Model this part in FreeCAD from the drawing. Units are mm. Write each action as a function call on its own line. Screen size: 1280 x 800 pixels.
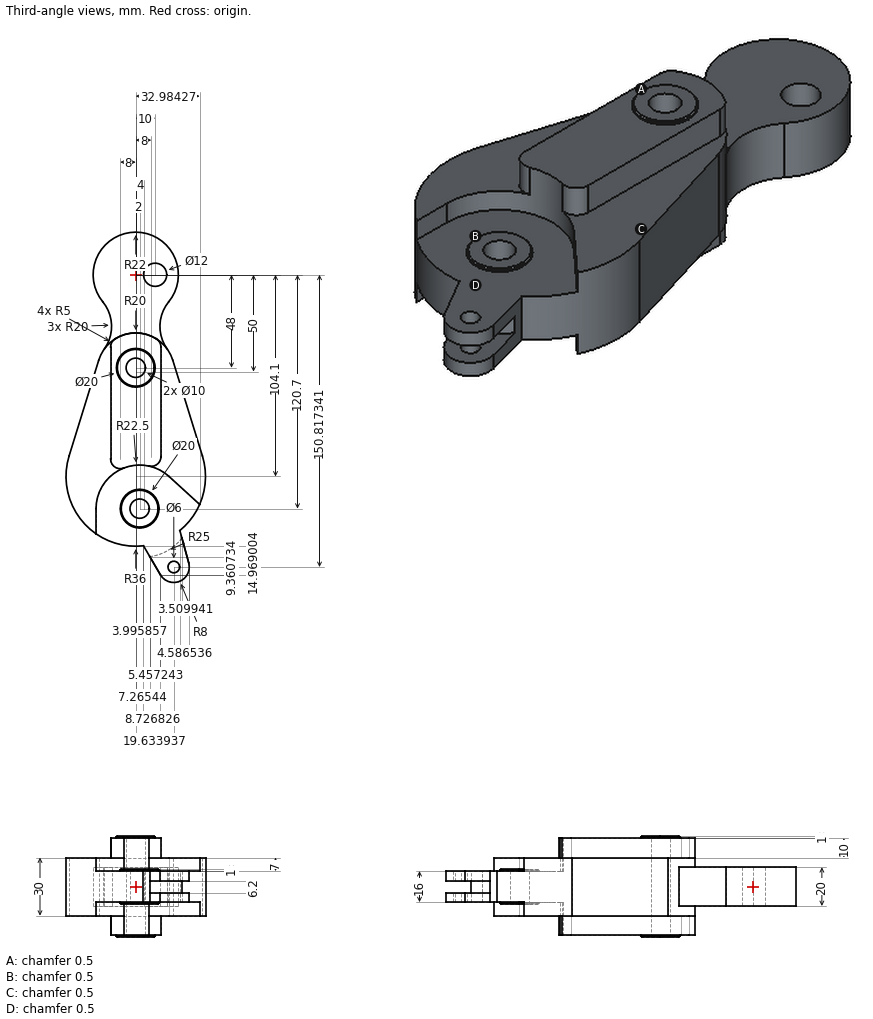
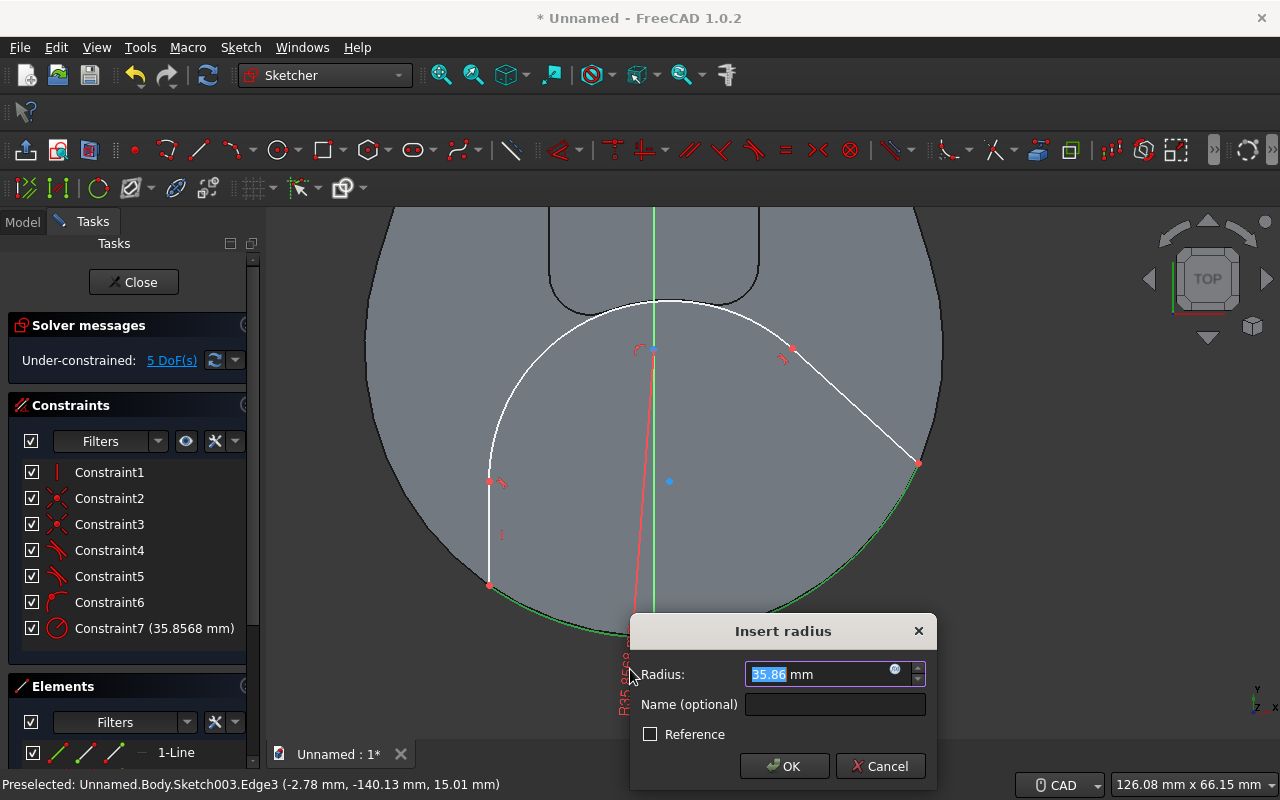
text(36)
key(Return)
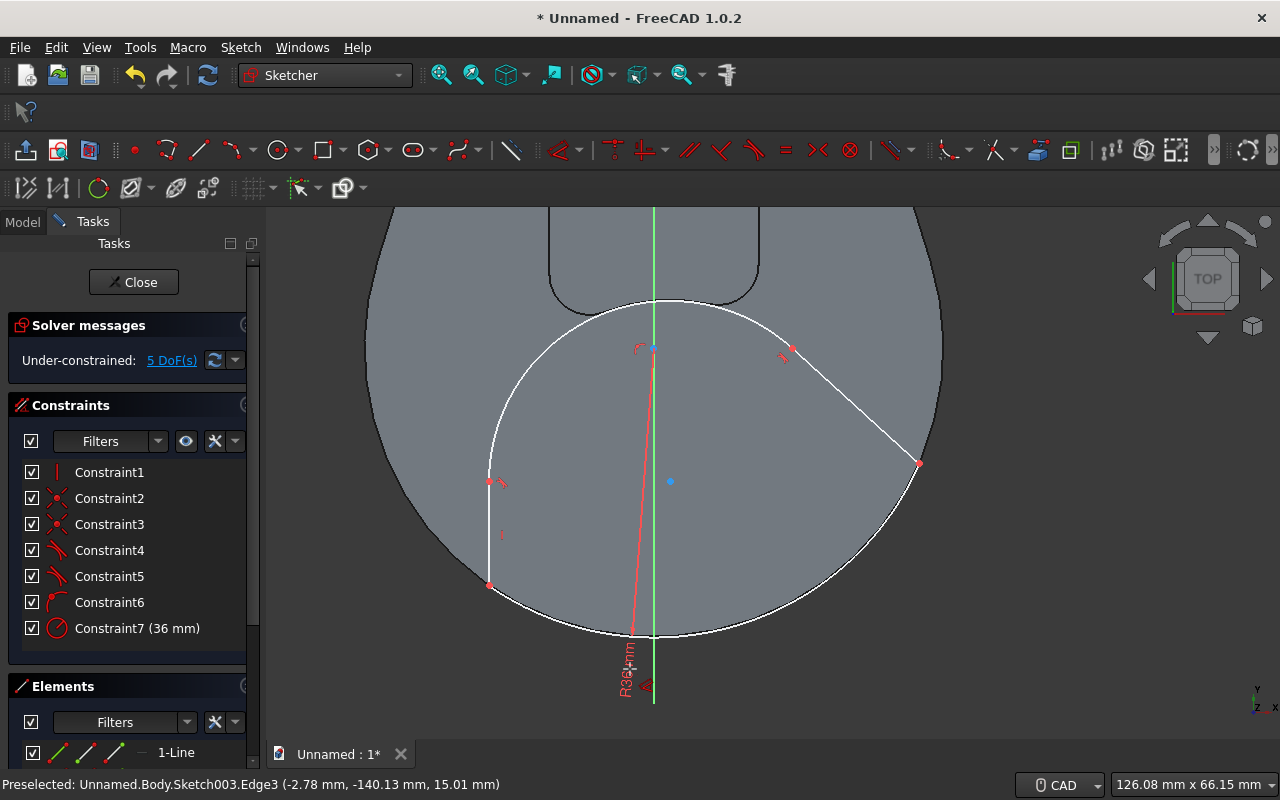
click(678, 301)
click(679, 269)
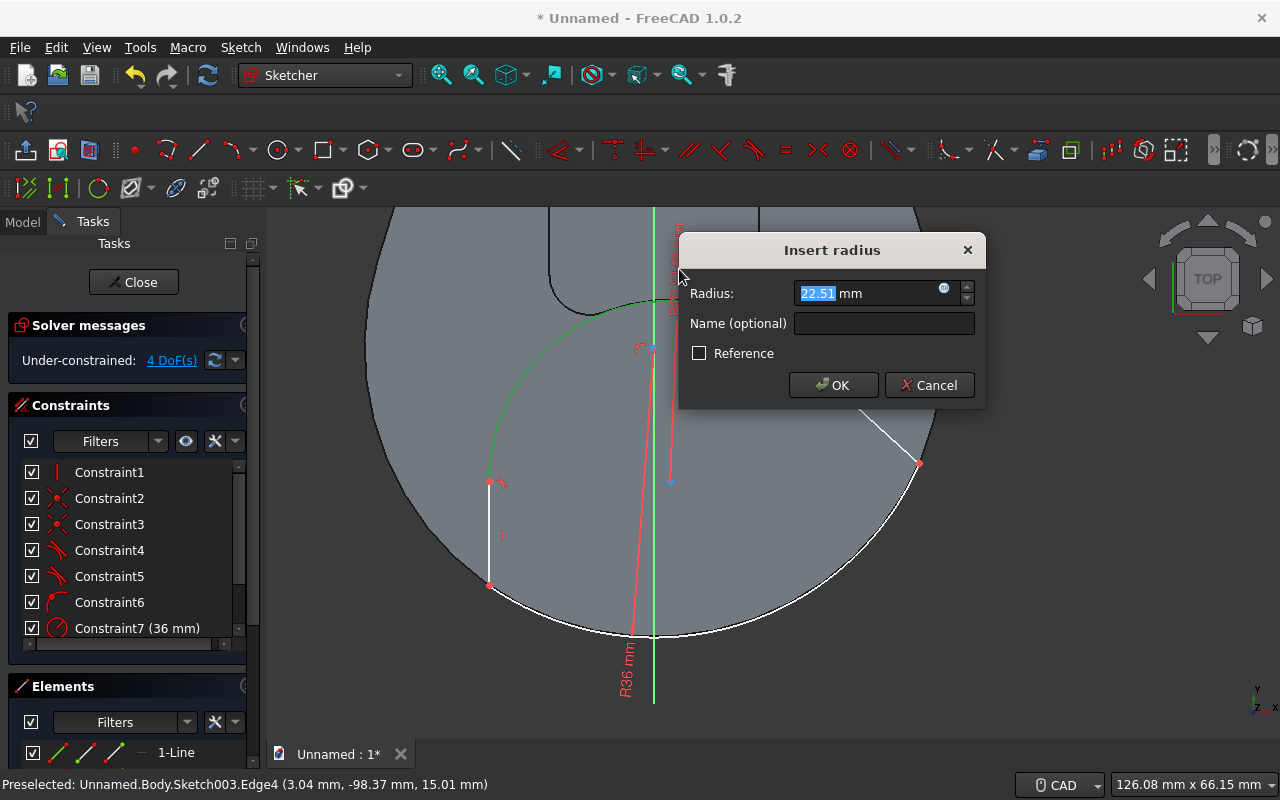
text(22.5)
key(Return)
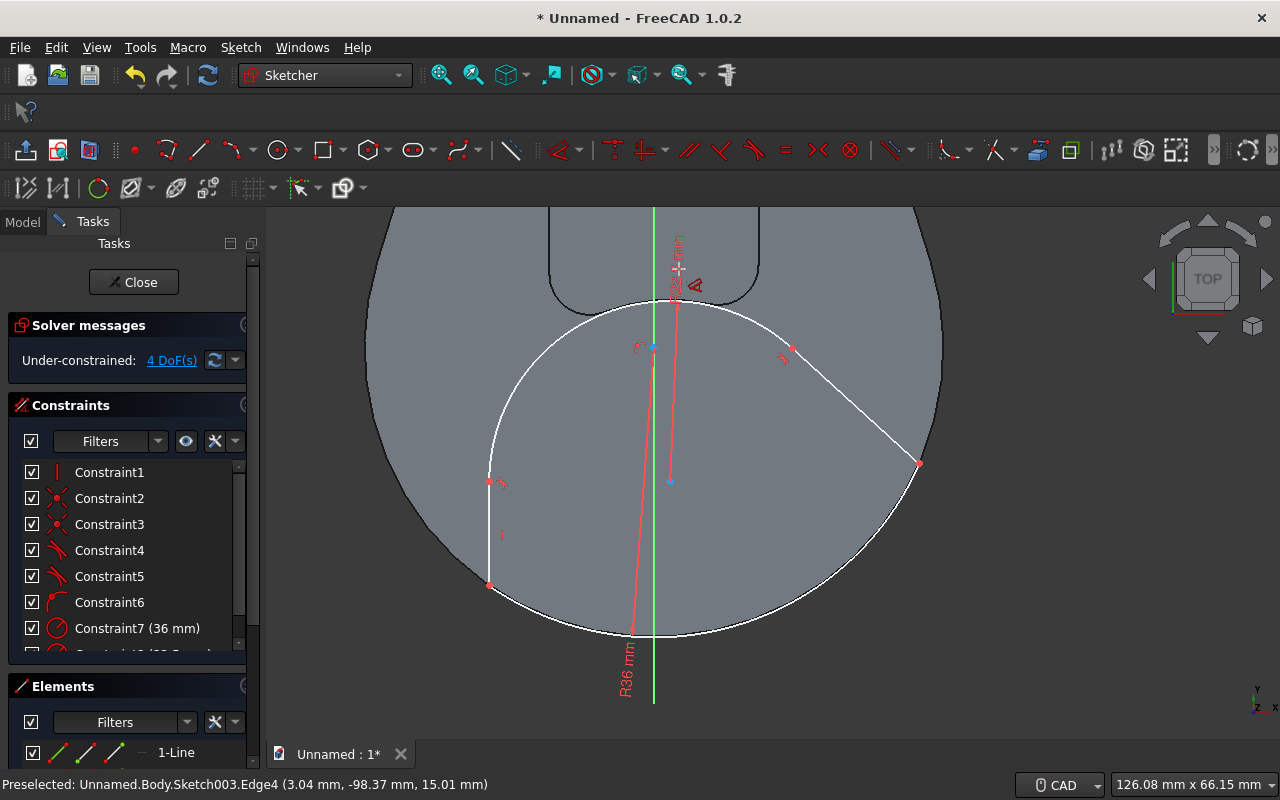
scroll(670, 482, up, 5)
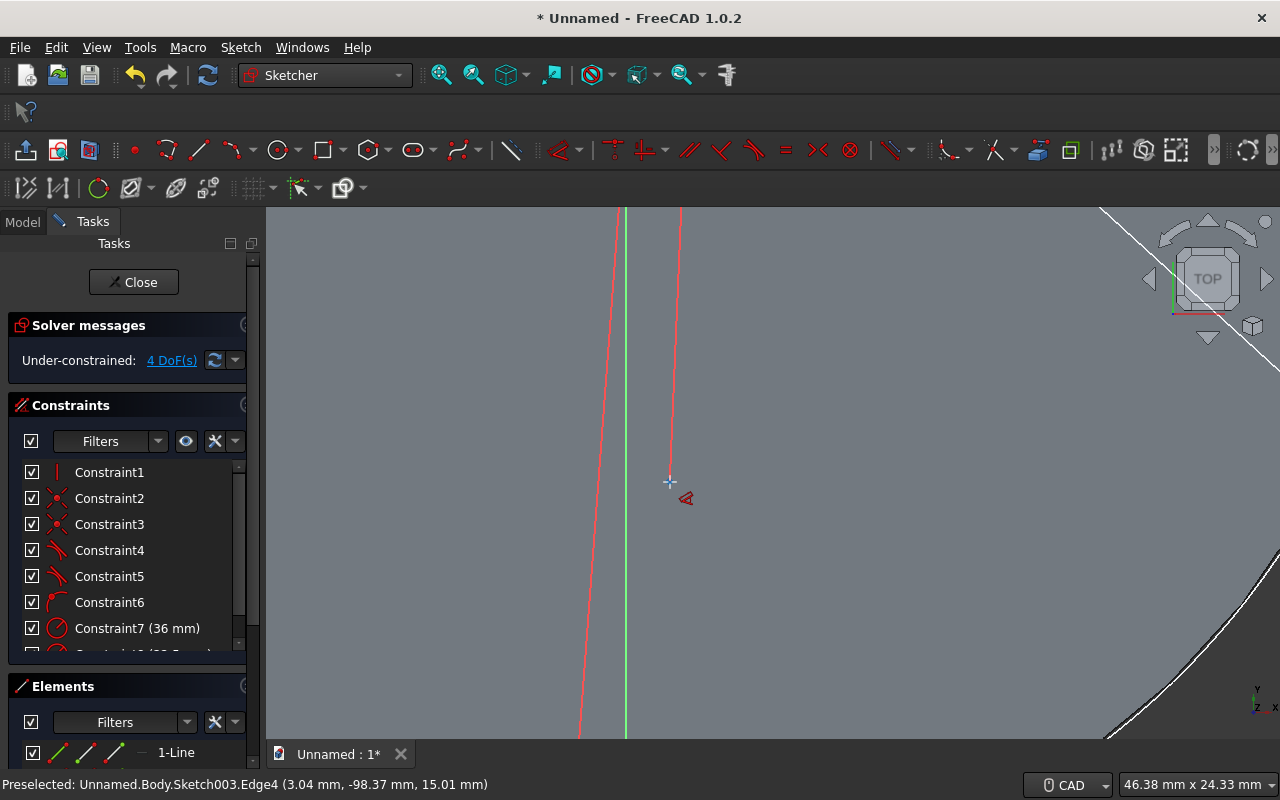
click(670, 481)
click(648, 515)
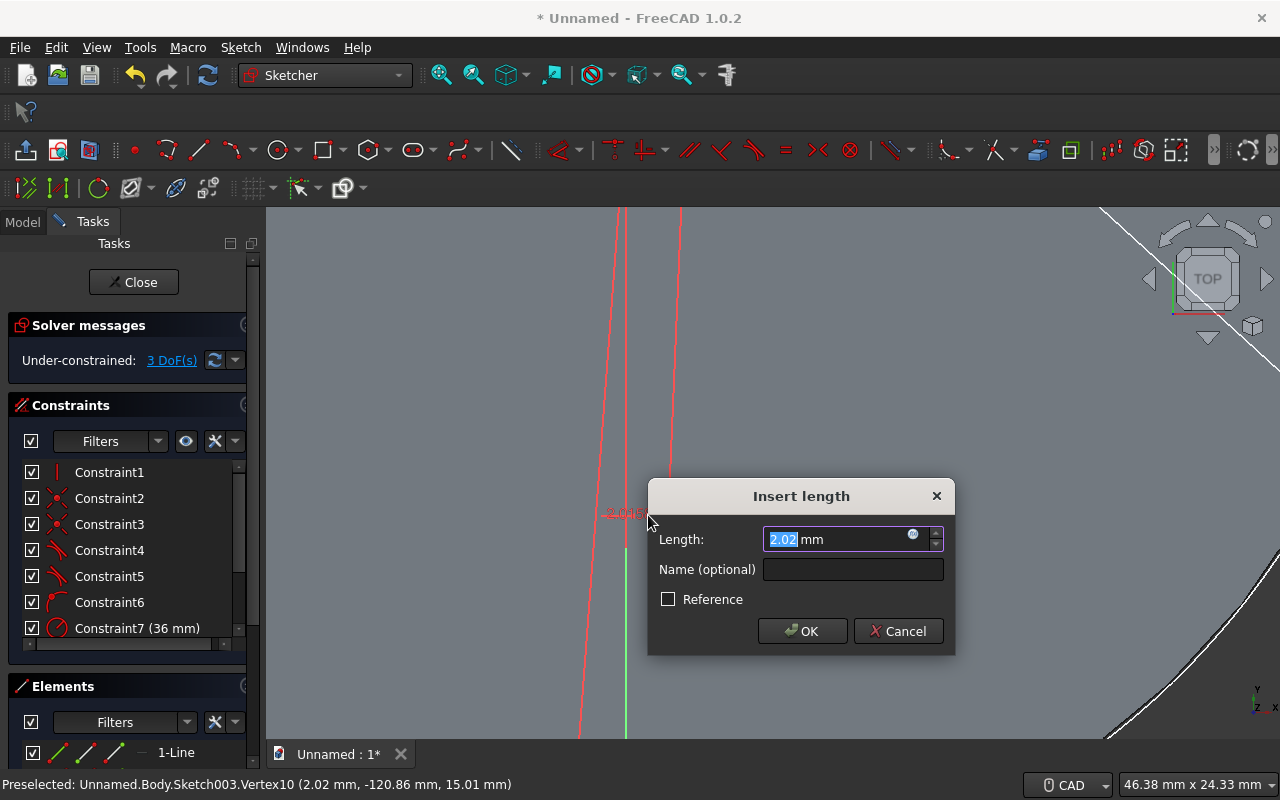
text(2)
key(Return)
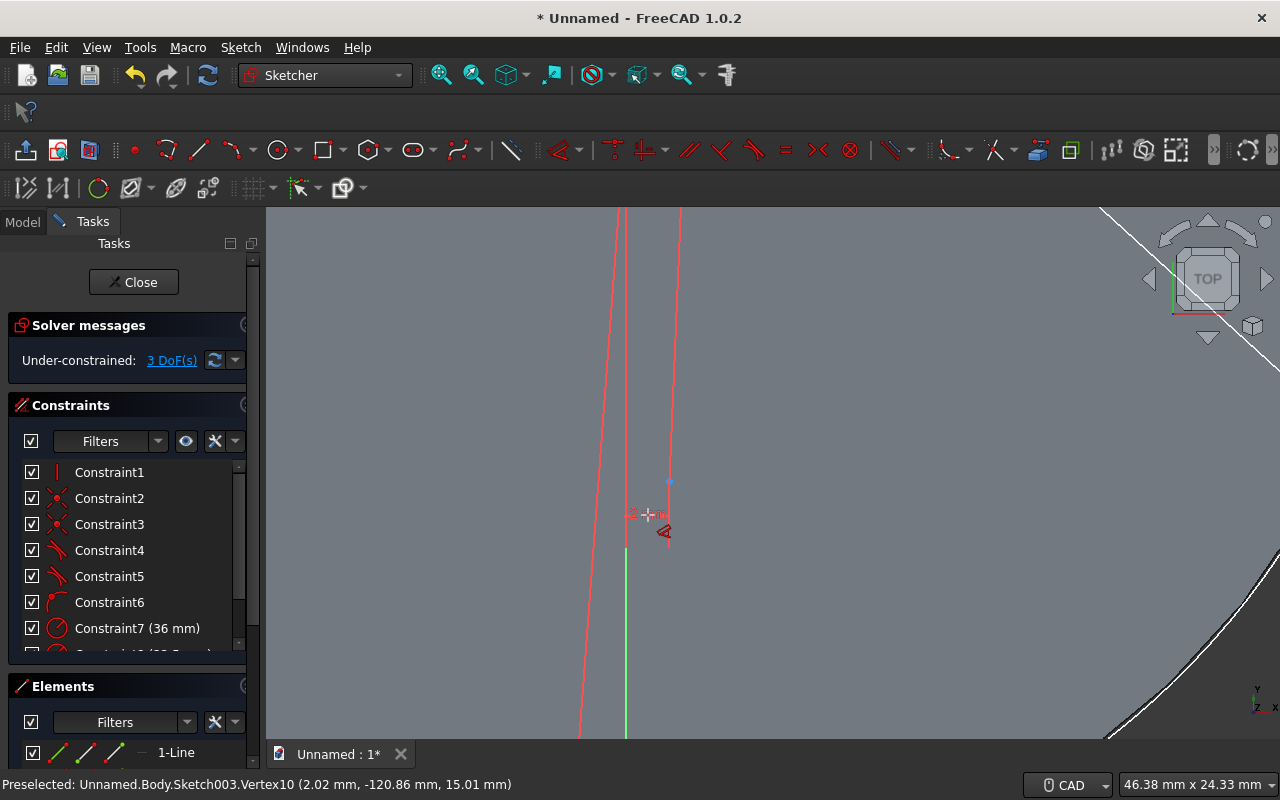
scroll(671, 487, down, 5)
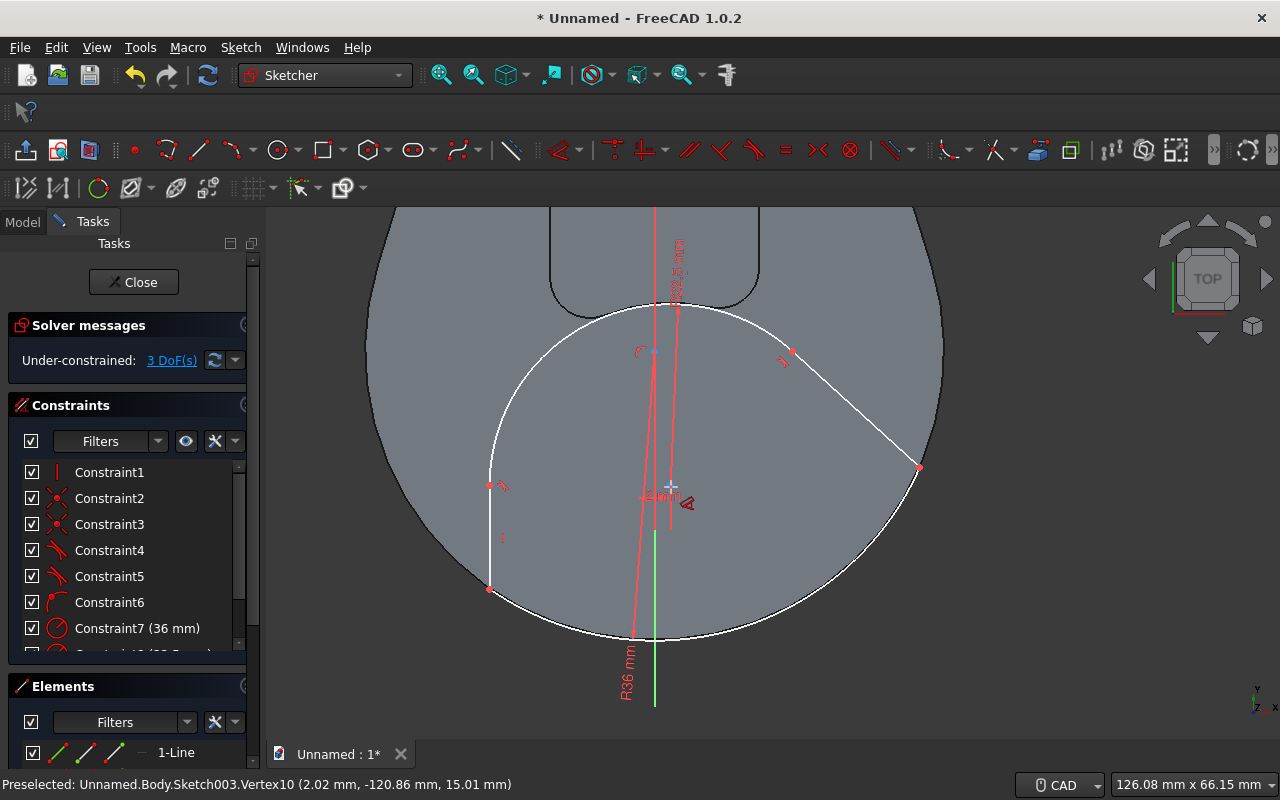
click(490, 485)
click(456, 360)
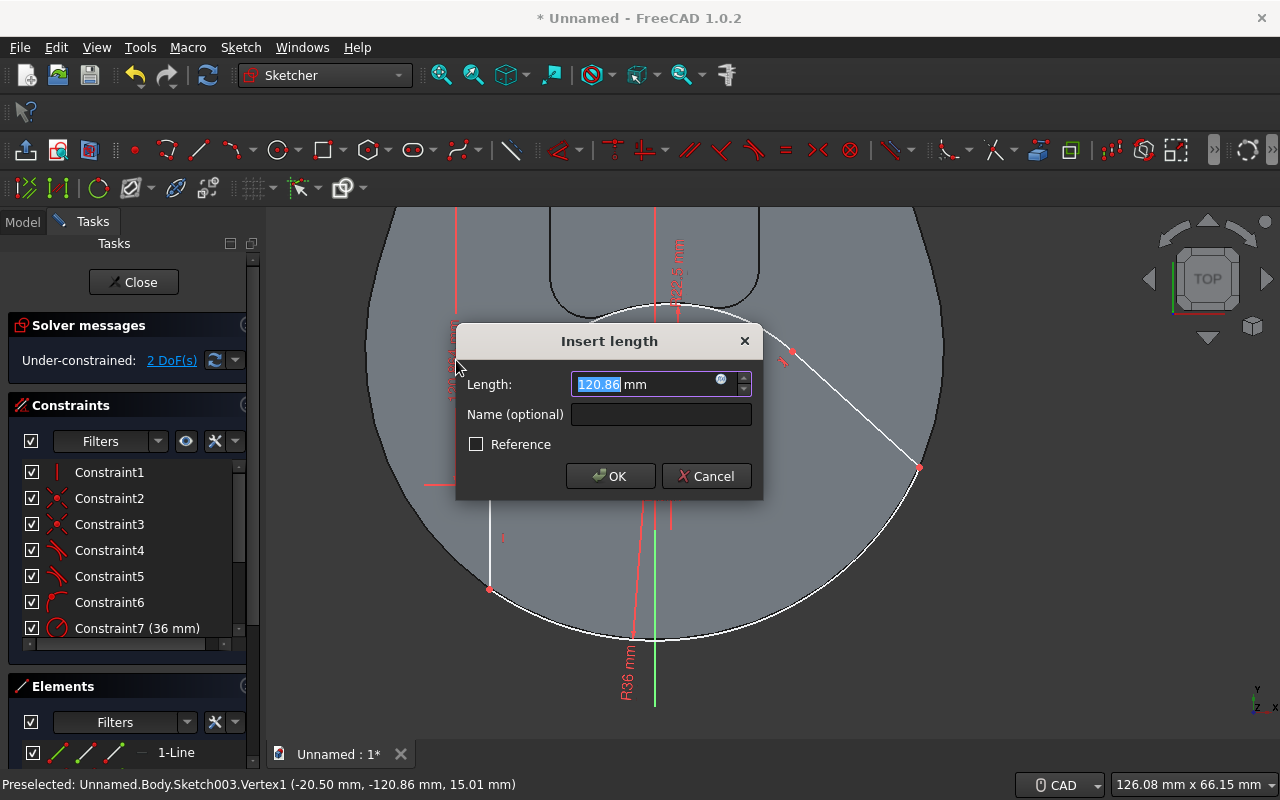
text(120.7)
key(Return)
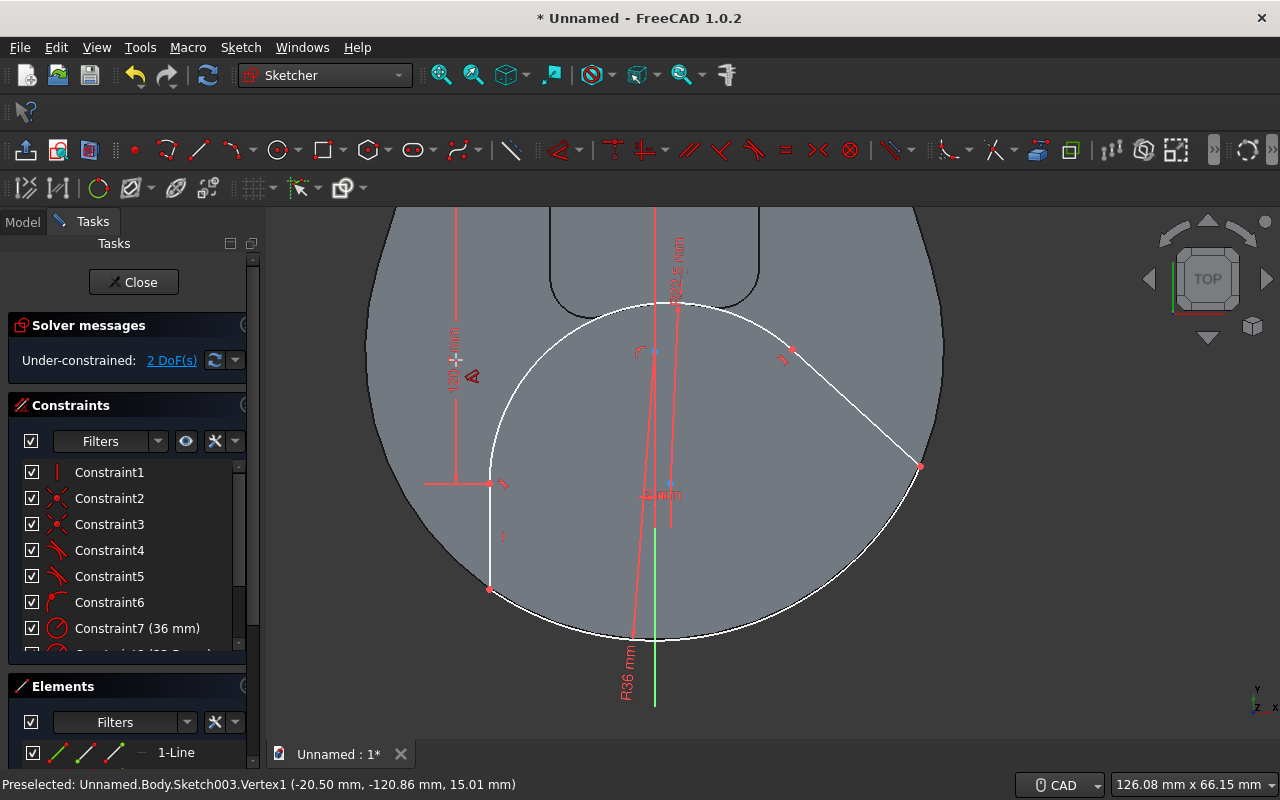
click(655, 351)
click(621, 293)